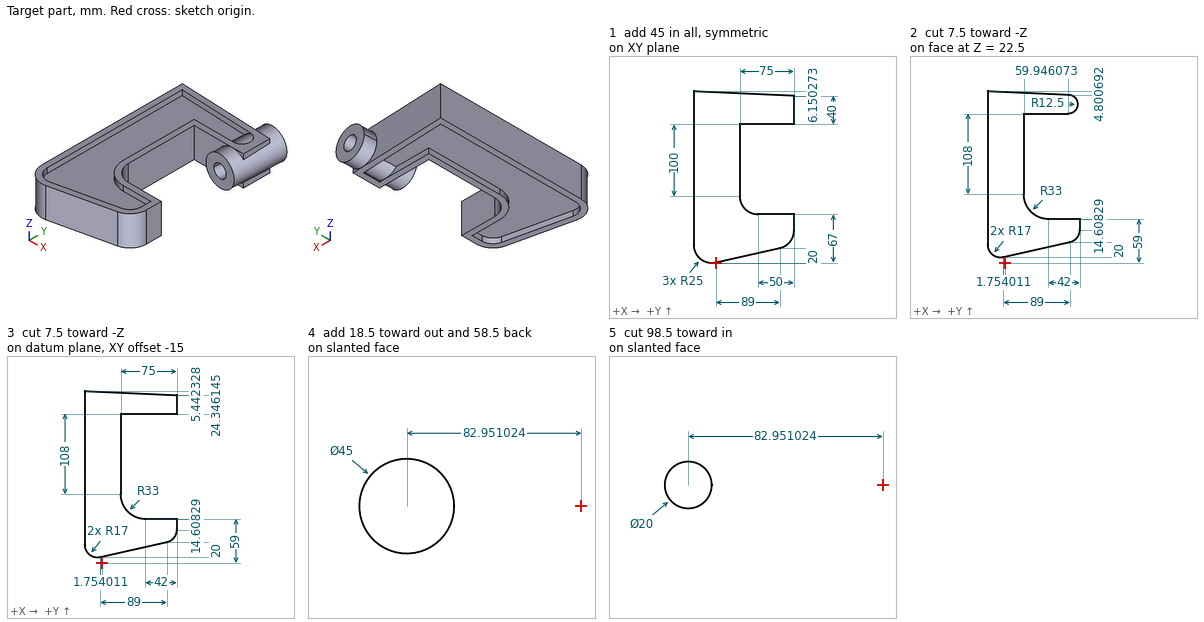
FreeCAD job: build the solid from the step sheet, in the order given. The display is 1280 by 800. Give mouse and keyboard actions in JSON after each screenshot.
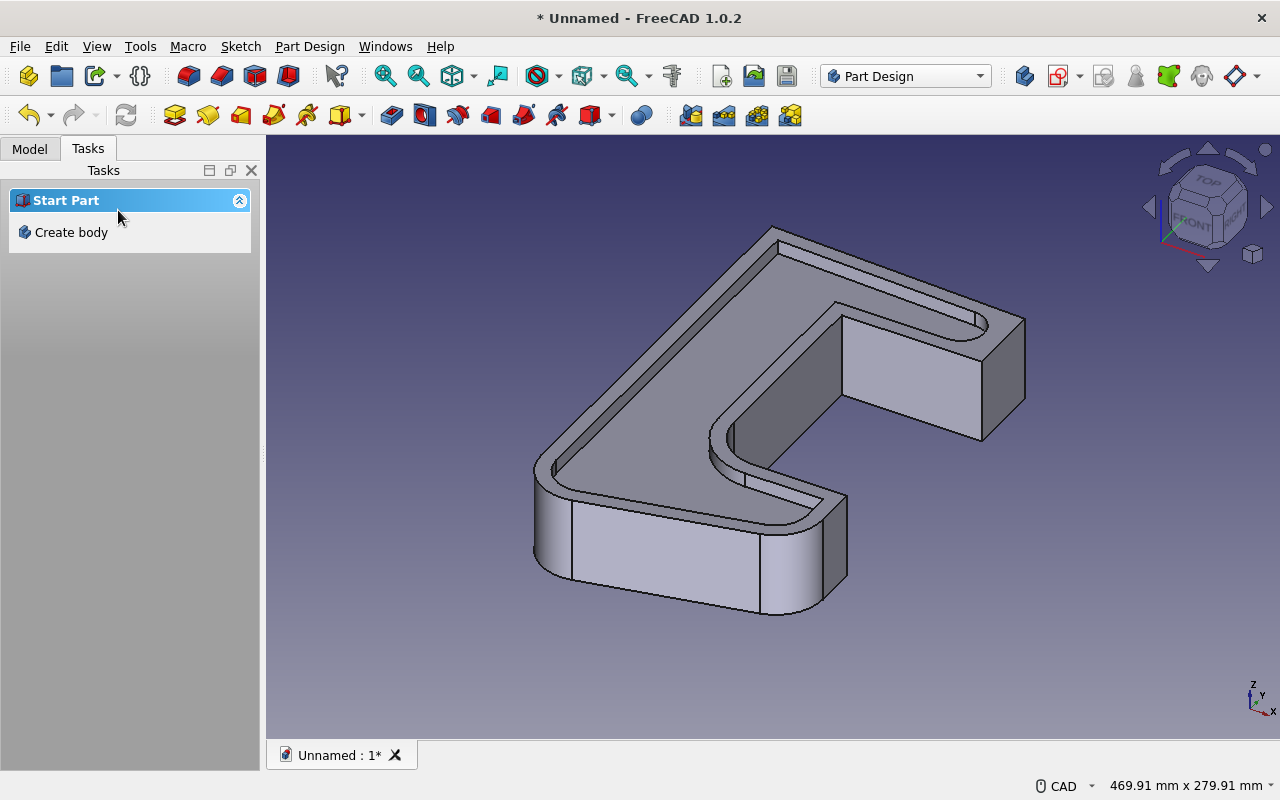
{"action": "left_click", "coordinate": [30, 148]}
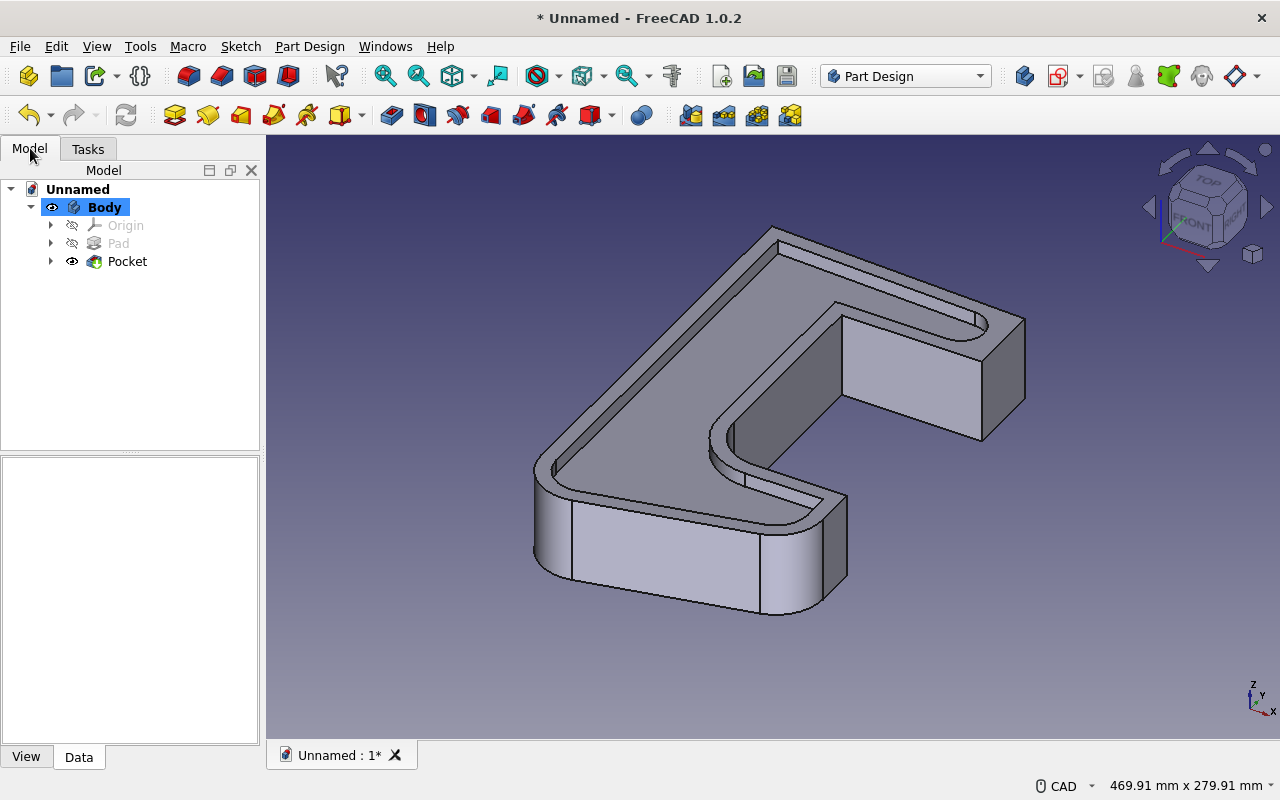
{"action": "left_click", "coordinate": [51, 225]}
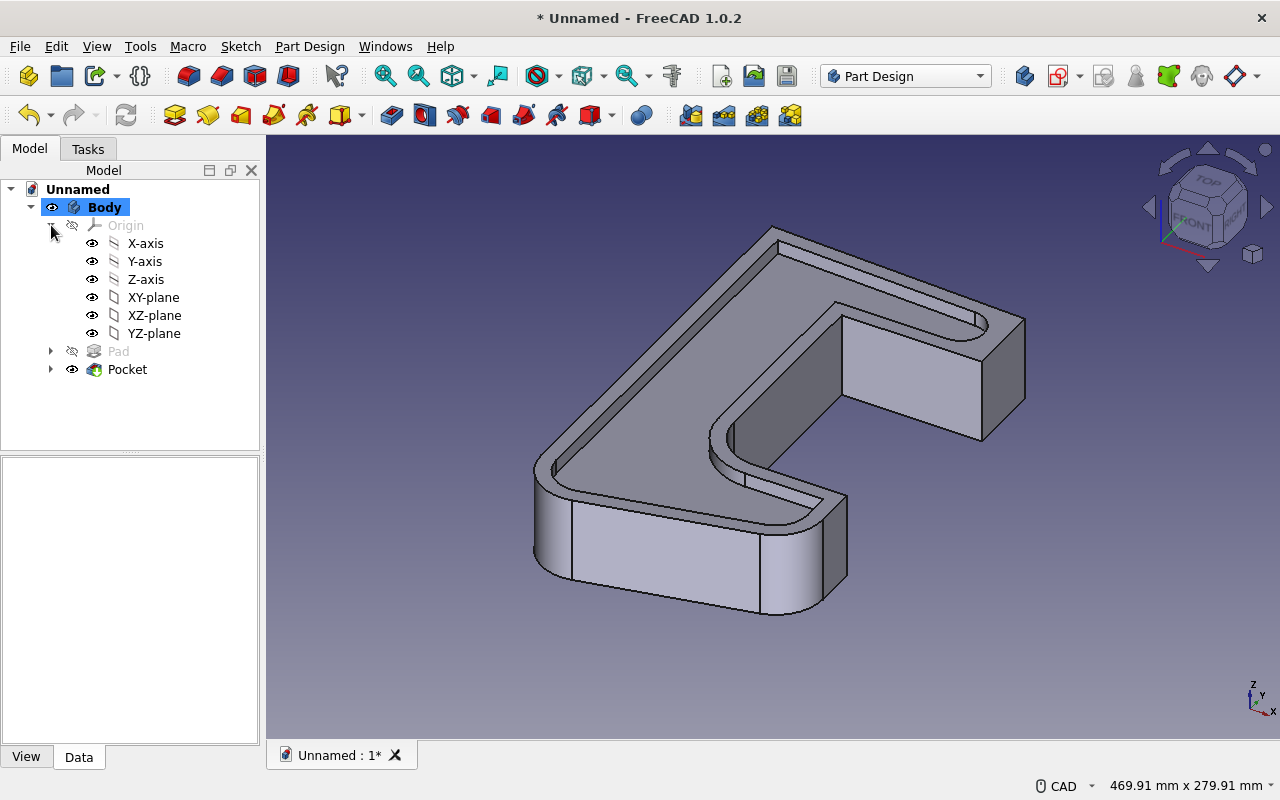
{"action": "left_click", "coordinate": [137, 297]}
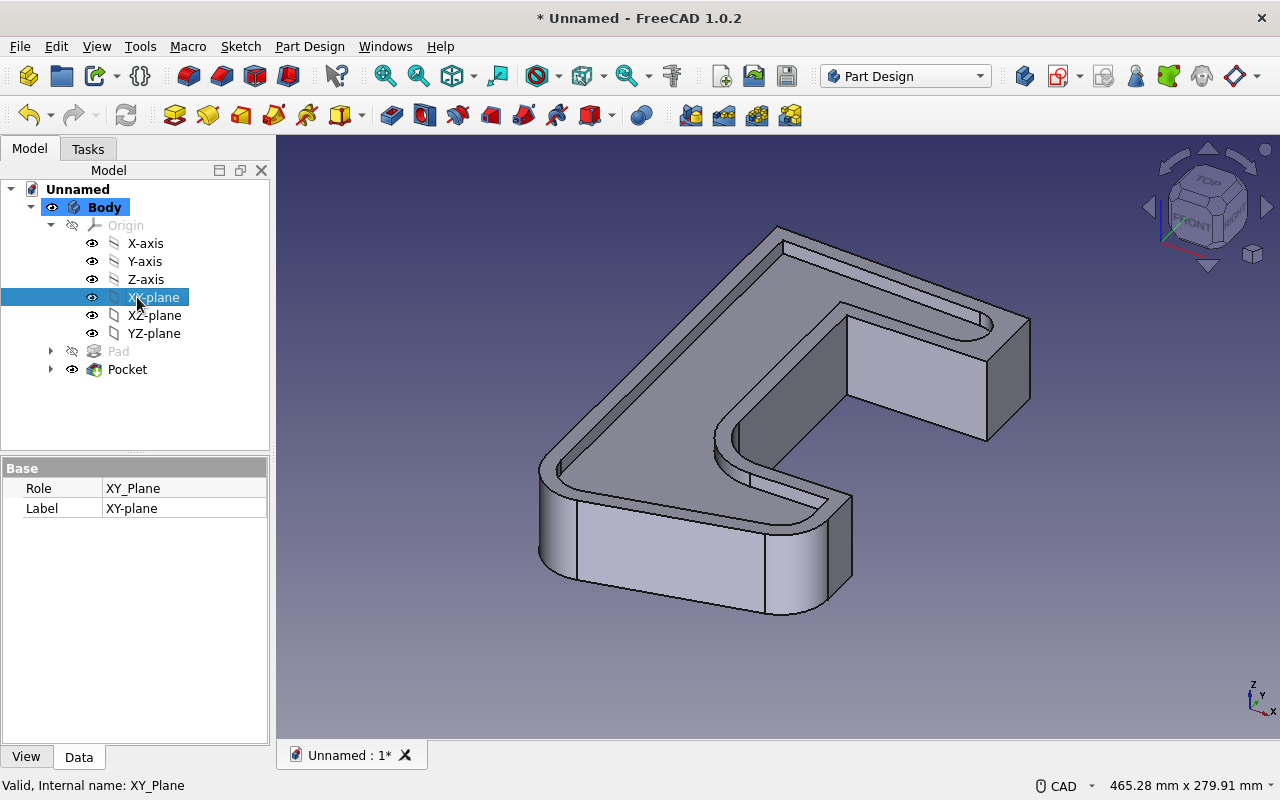
{"action": "left_click", "coordinate": [1234, 76]}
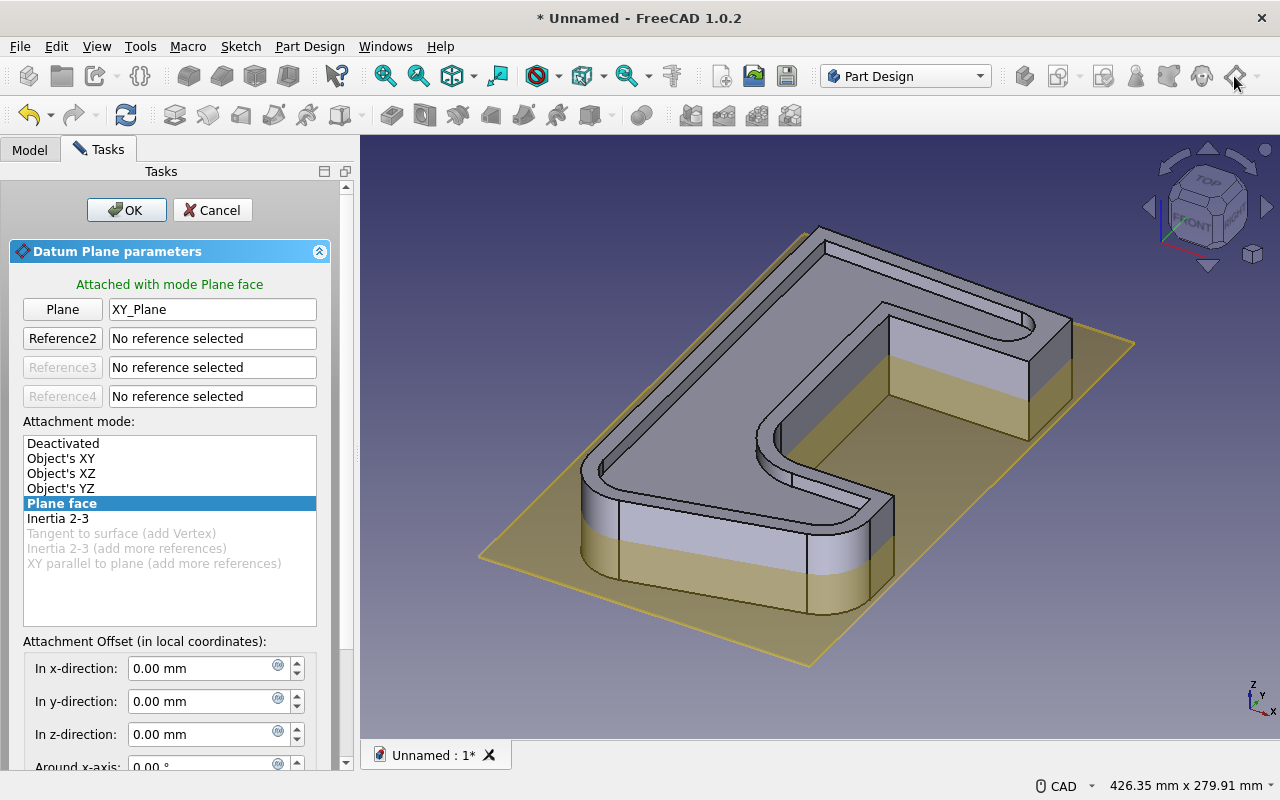
{"action": "triple_click", "coordinate": [210, 734]}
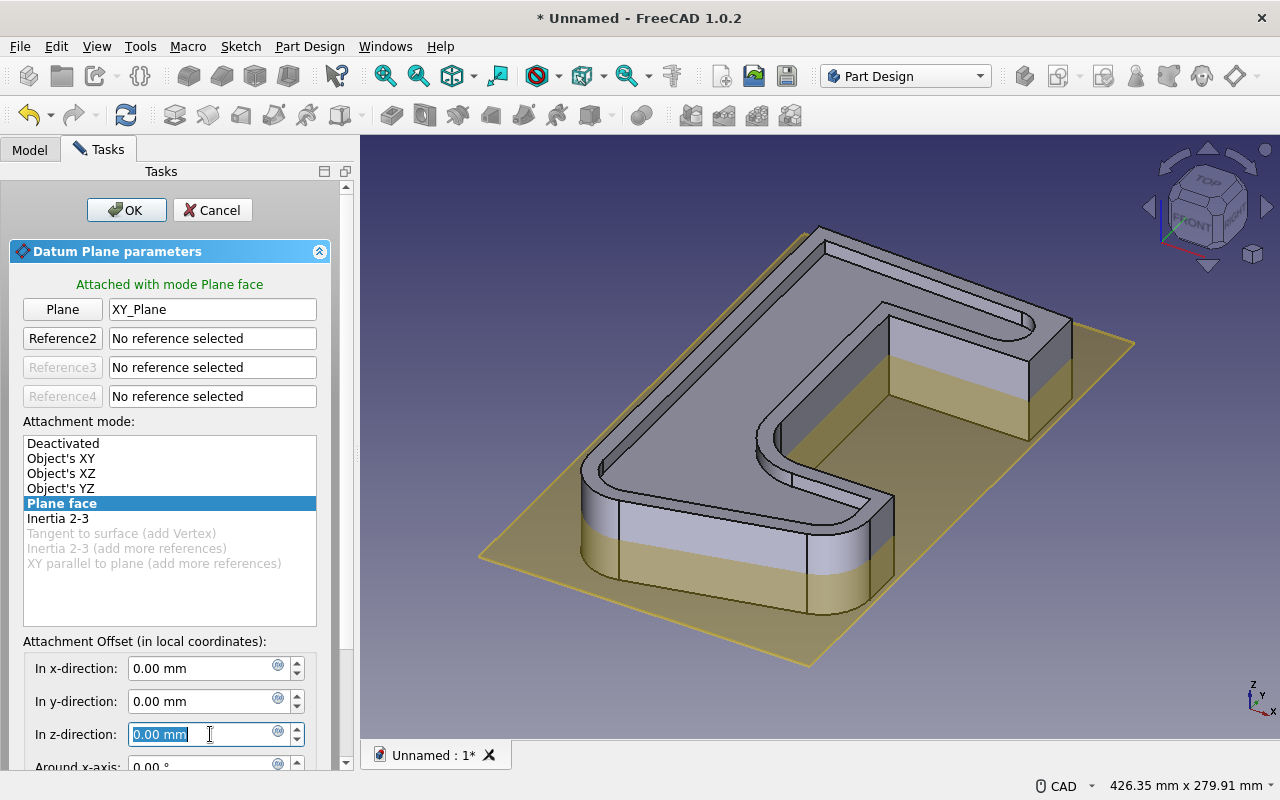
{"action": "type", "text": "-15"}
{"action": "key", "text": "Tab"}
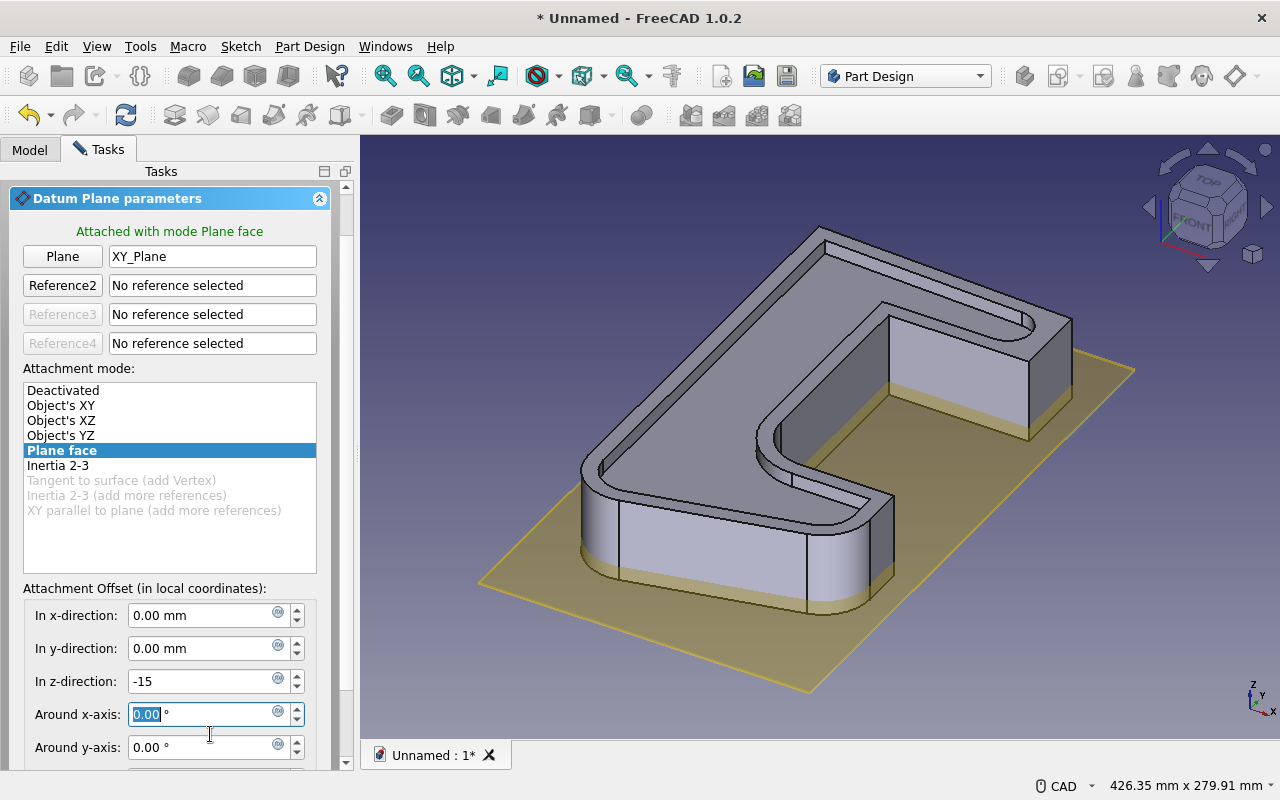
{"action": "scroll", "coordinate": [346, 476], "scroll_direction": "up", "scroll_amount": 2}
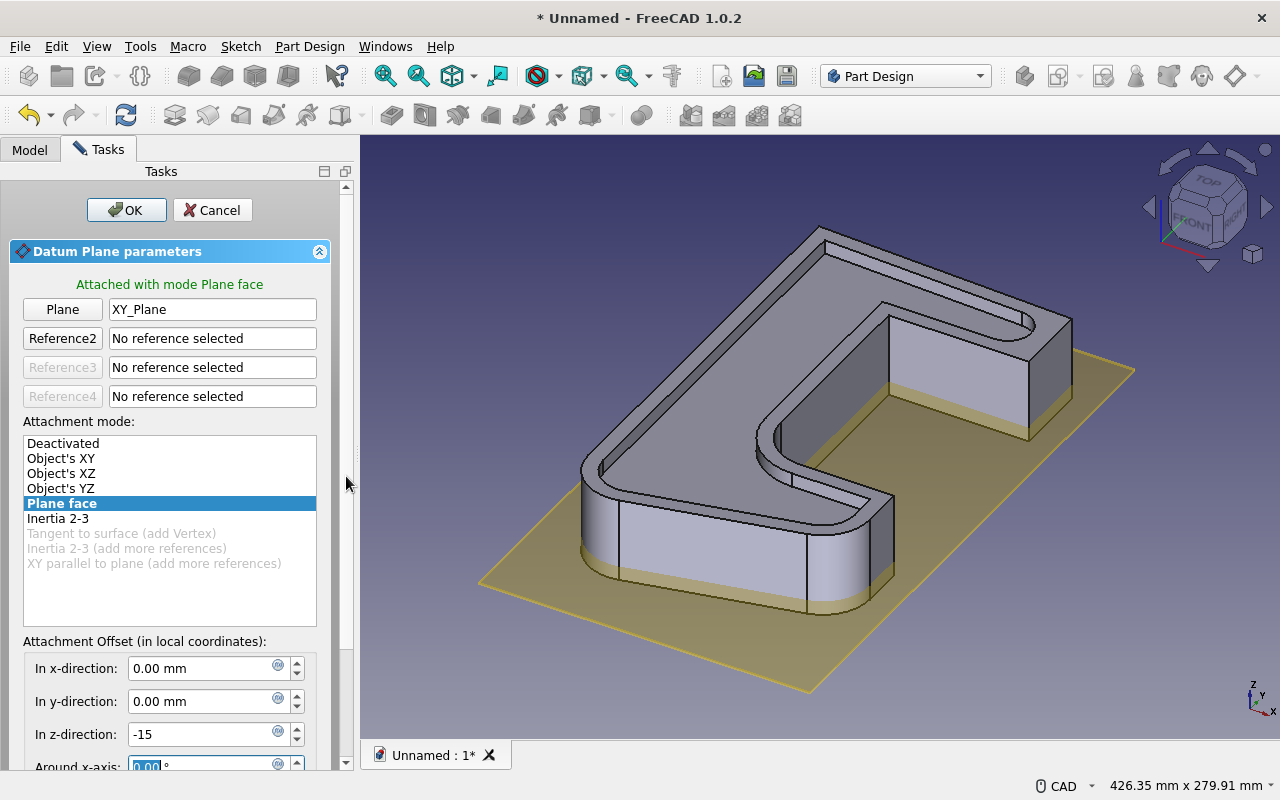
{"action": "left_click", "coordinate": [127, 210]}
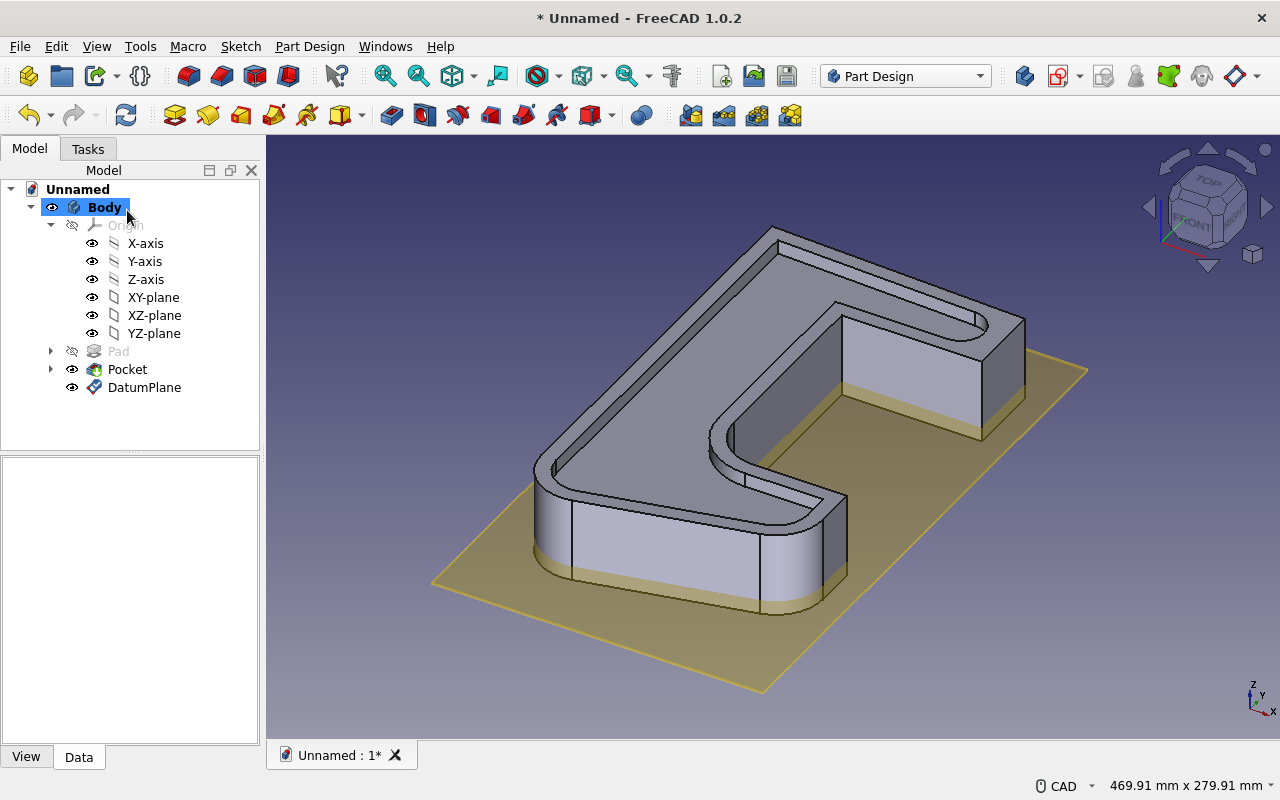
{"action": "left_click", "coordinate": [117, 387]}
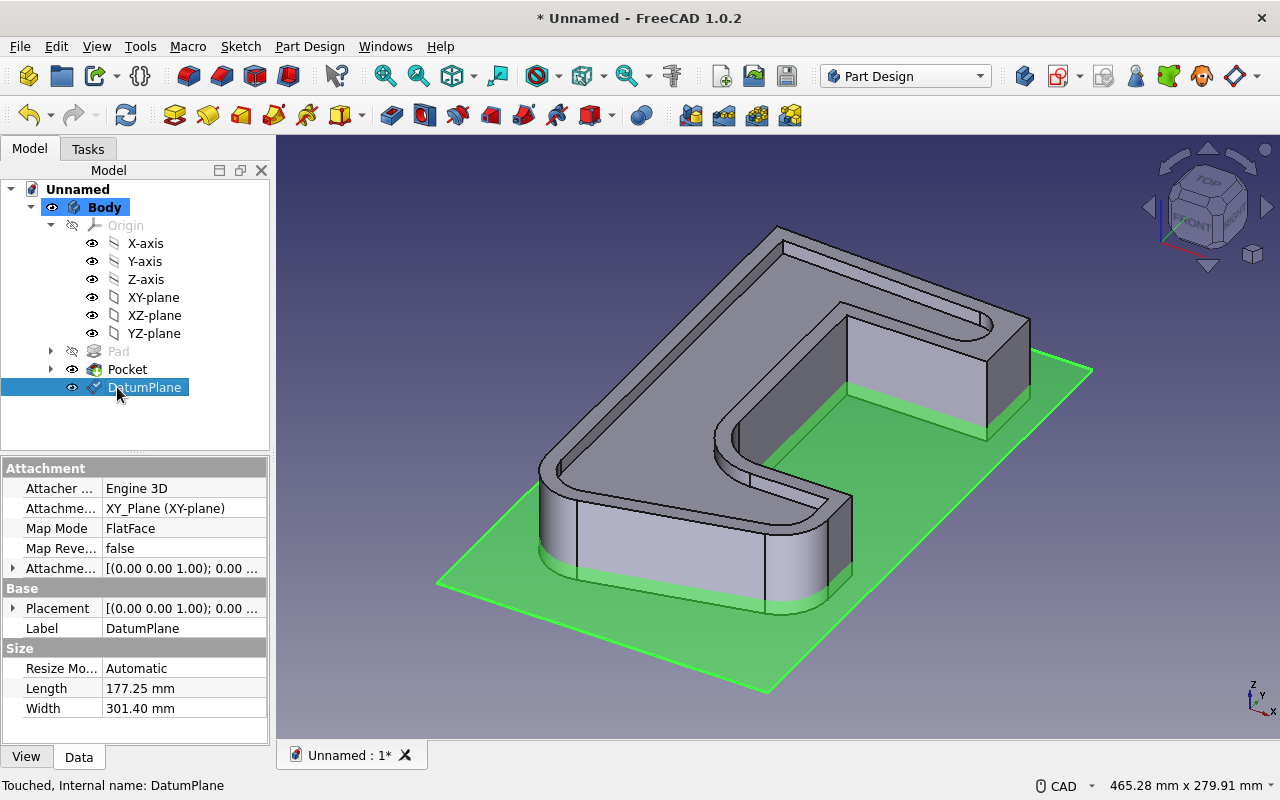
{"action": "left_click", "coordinate": [1058, 76]}